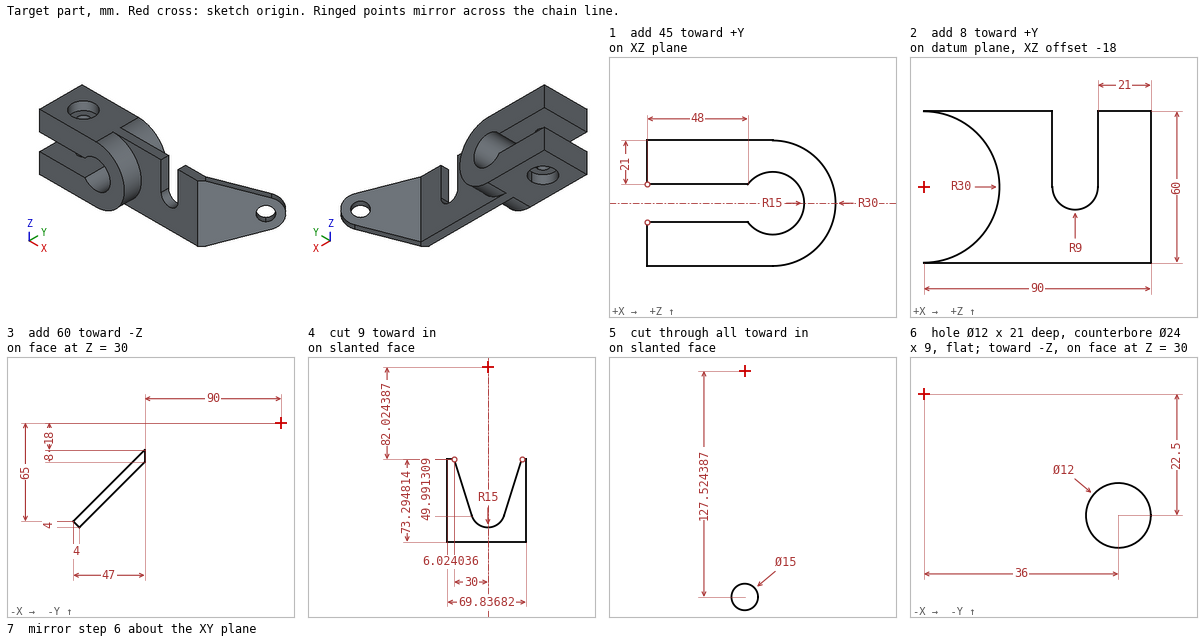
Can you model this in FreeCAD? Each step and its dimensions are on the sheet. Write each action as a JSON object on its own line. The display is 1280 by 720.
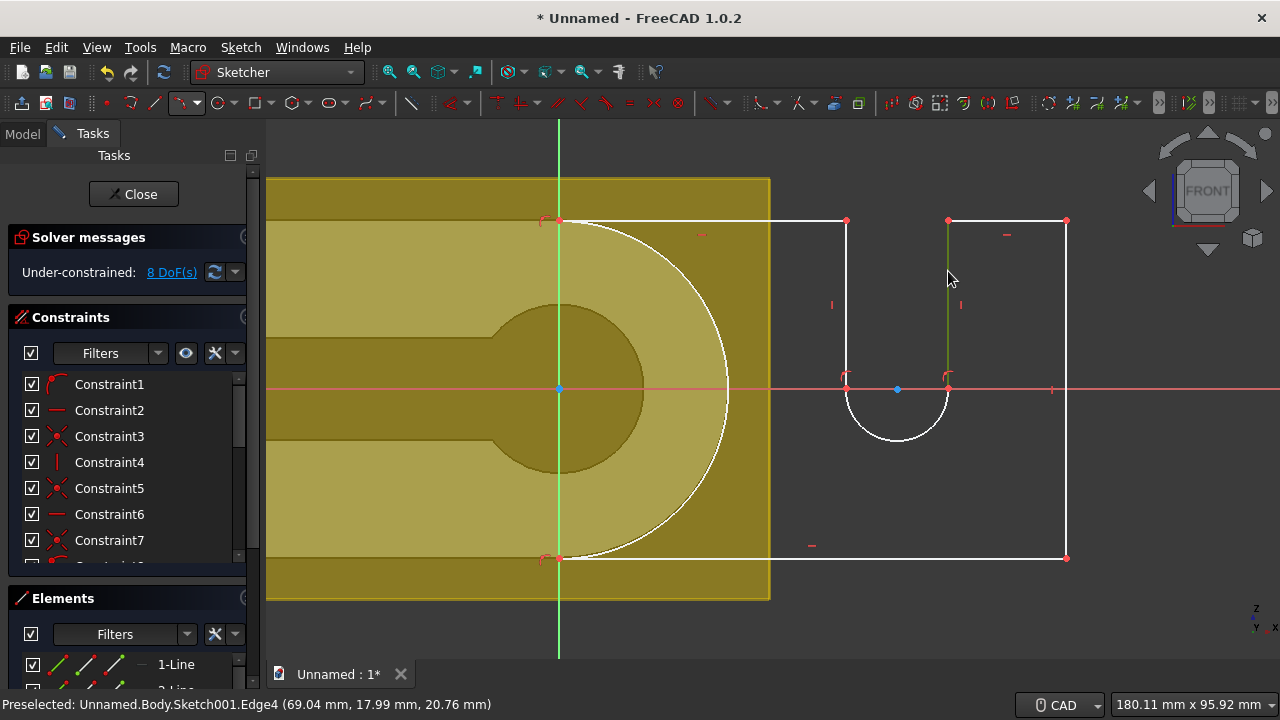
{"action": "left_click", "coordinate": [867, 431]}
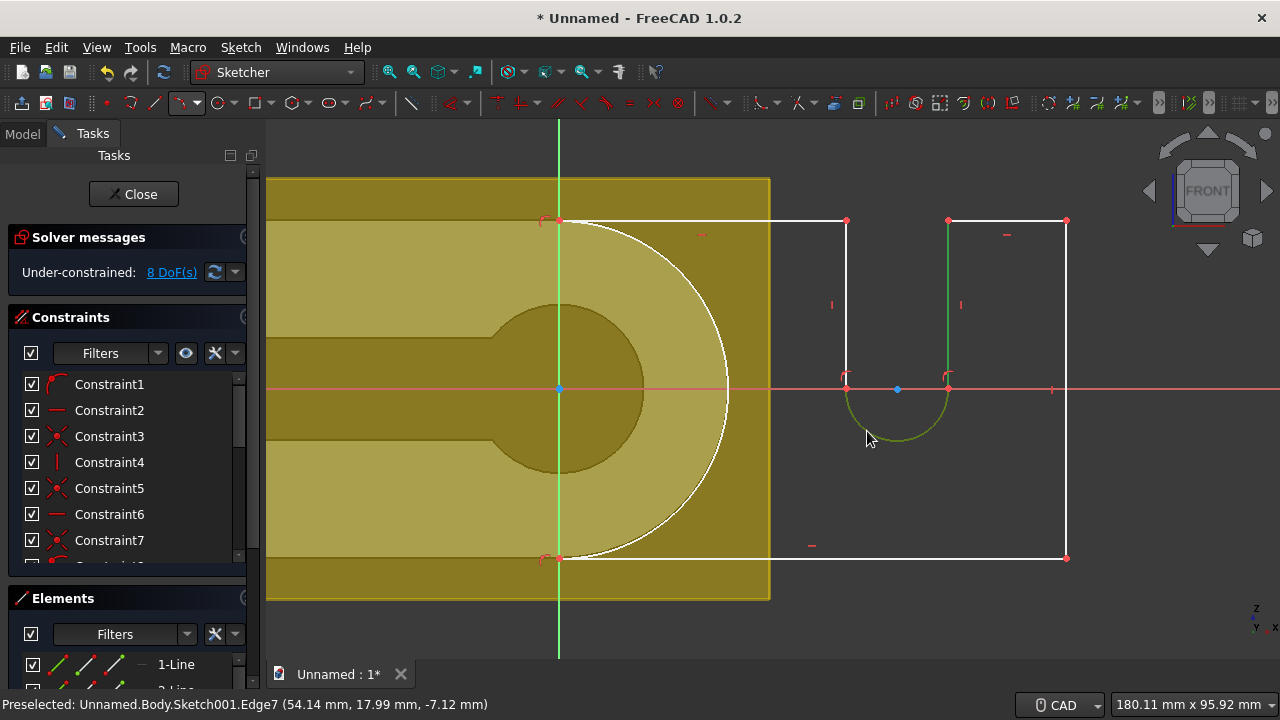
{"action": "left_click", "coordinate": [606, 104]}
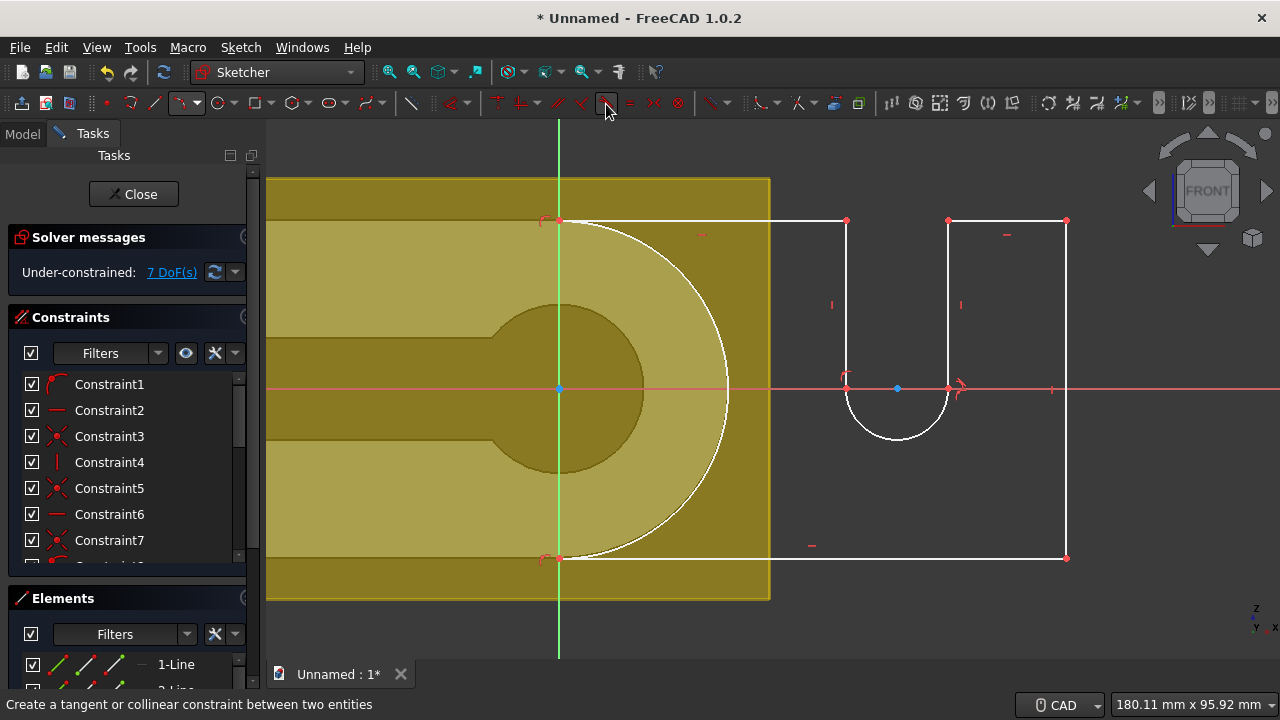
{"action": "left_click_drag", "start_coordinate": [549, 379], "coordinate": [569, 400]}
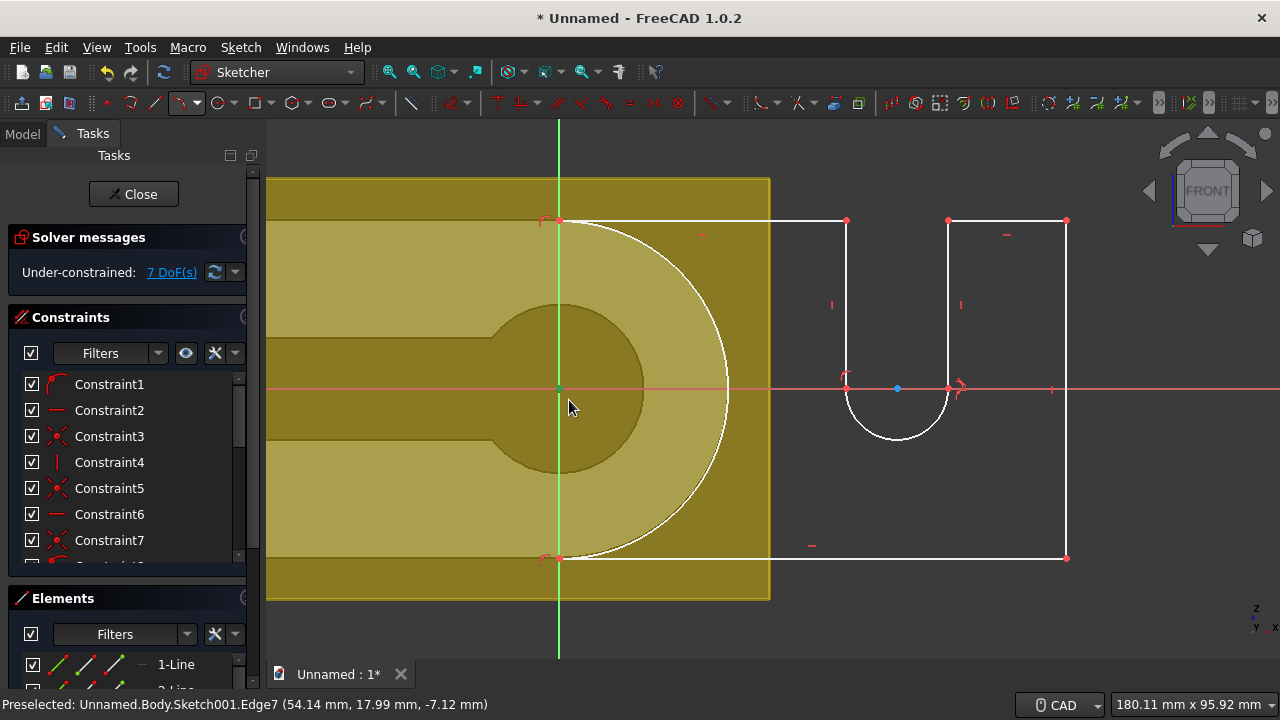
{"action": "left_click", "coordinate": [498, 104]}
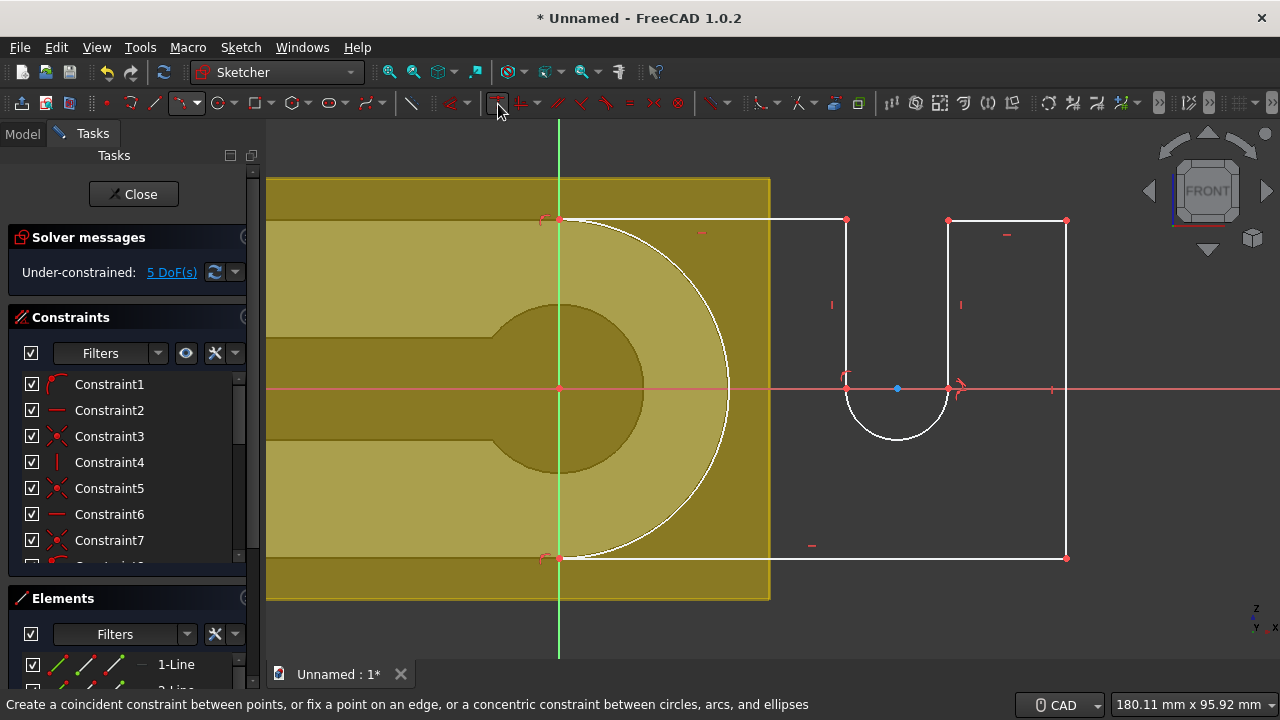
{"action": "left_click", "coordinate": [450, 104]}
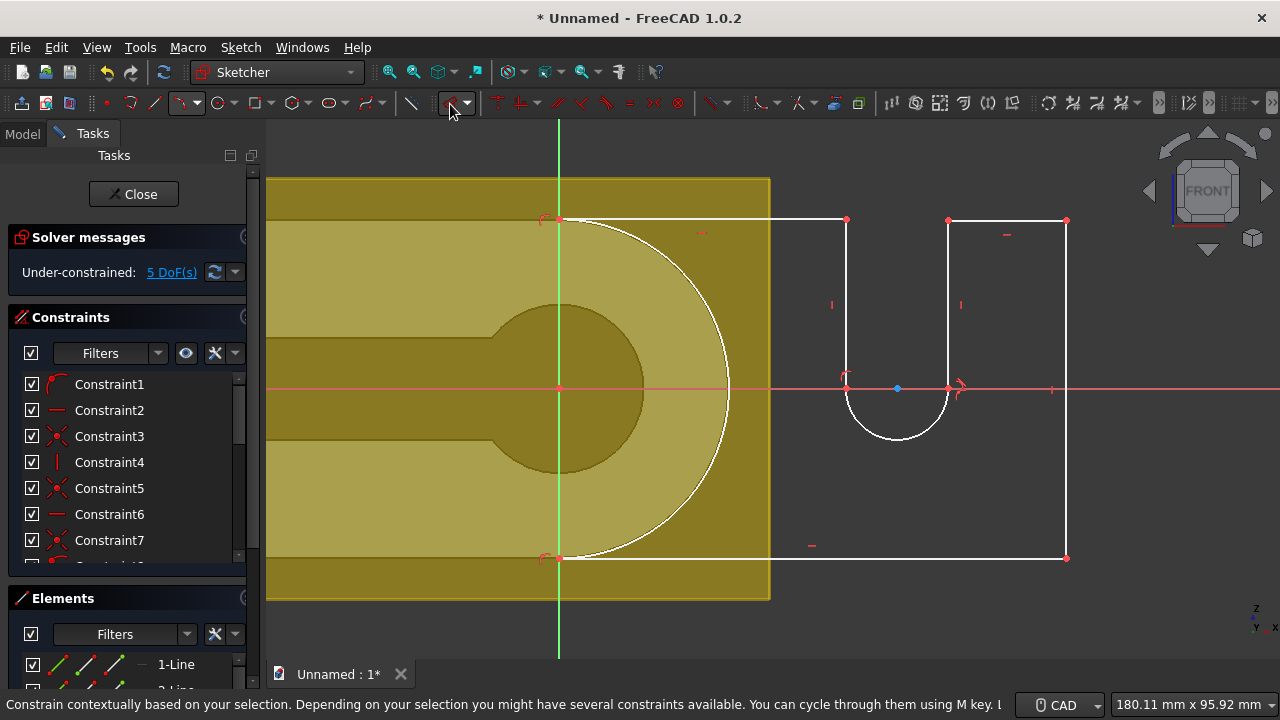
{"action": "left_click", "coordinate": [867, 430]}
{"action": "left_click", "coordinate": [848, 456]}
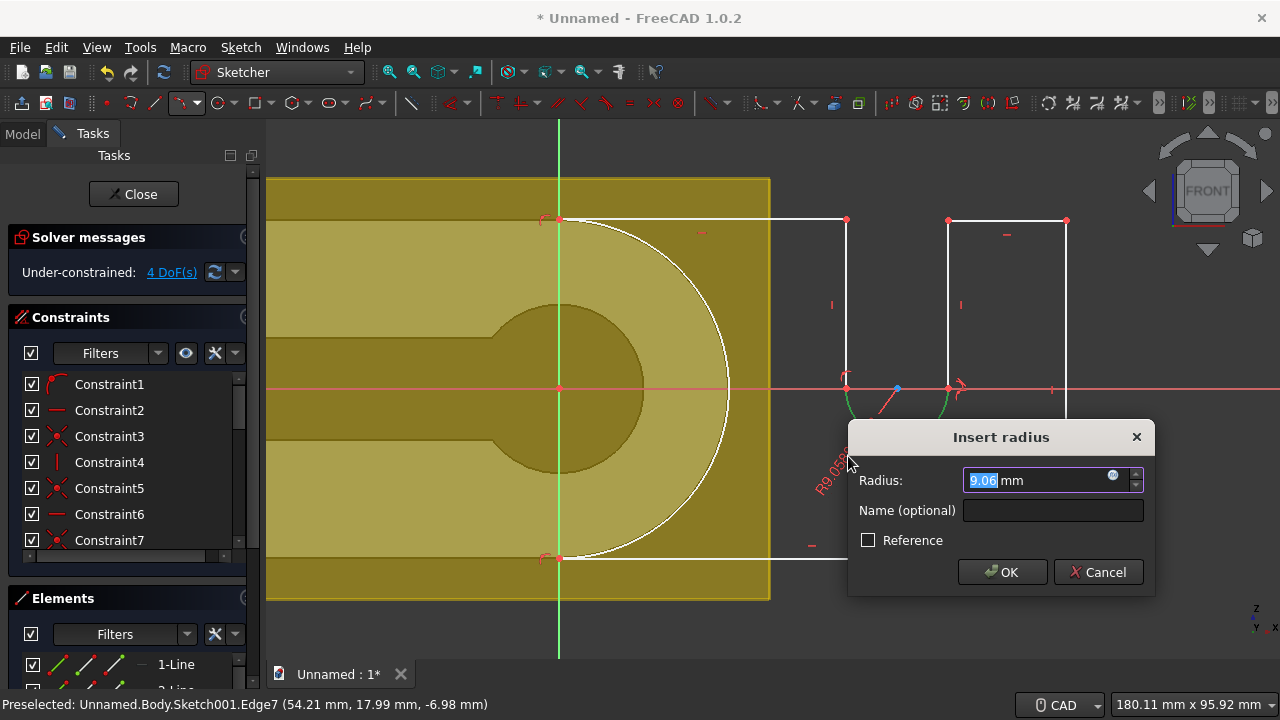
{"action": "type", "text": "9"}
{"action": "key", "text": "Return"}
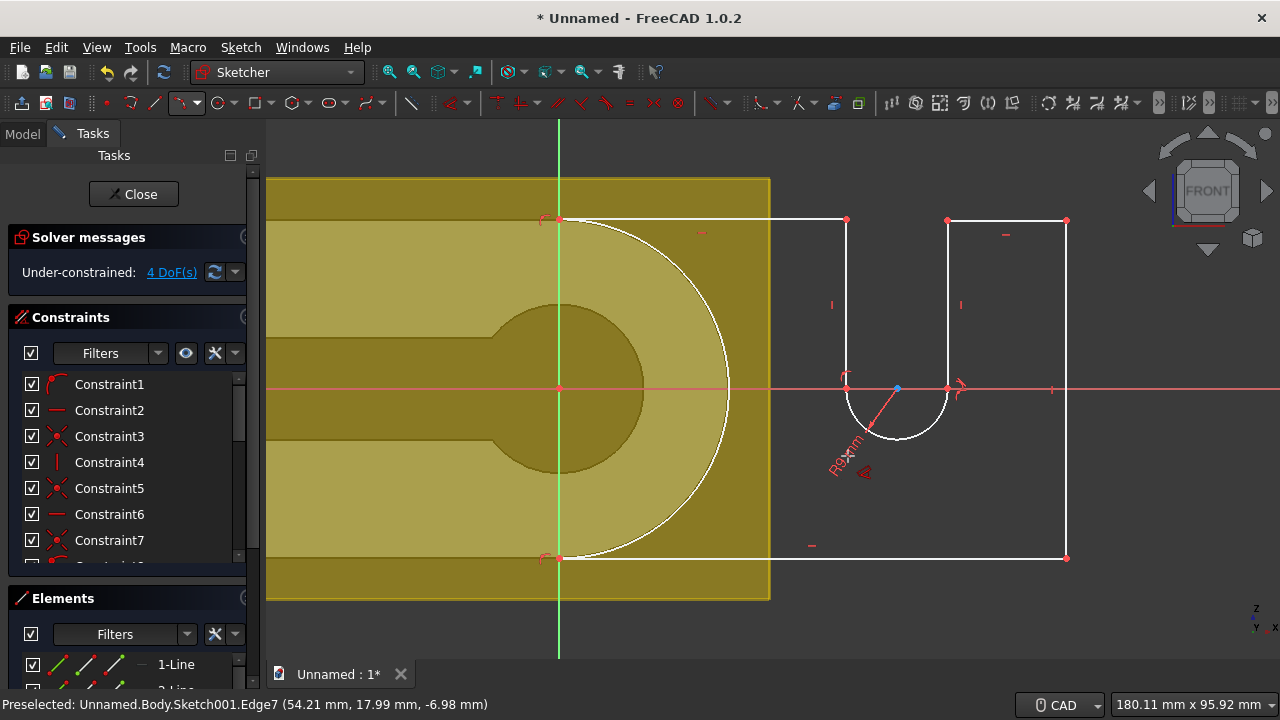
{"action": "left_click", "coordinate": [697, 489]}
{"action": "left_click", "coordinate": [723, 508]}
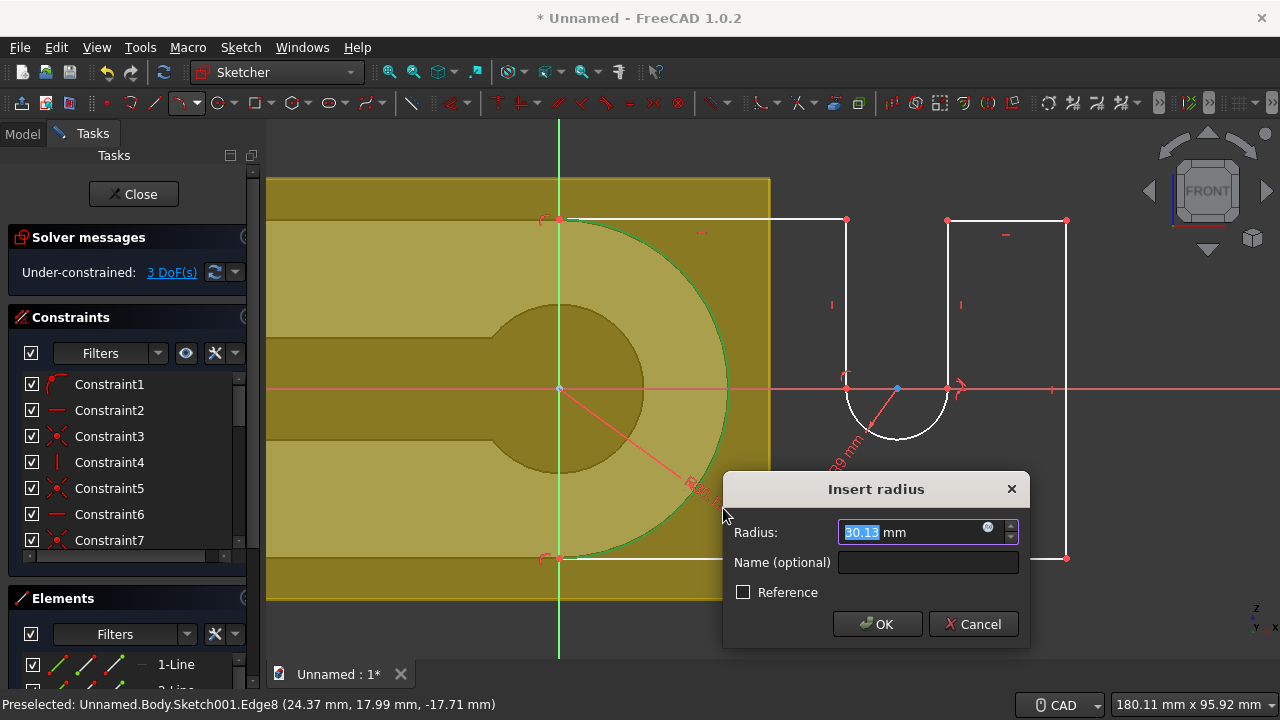
{"action": "type", "text": "30"}
{"action": "key", "text": "Return"}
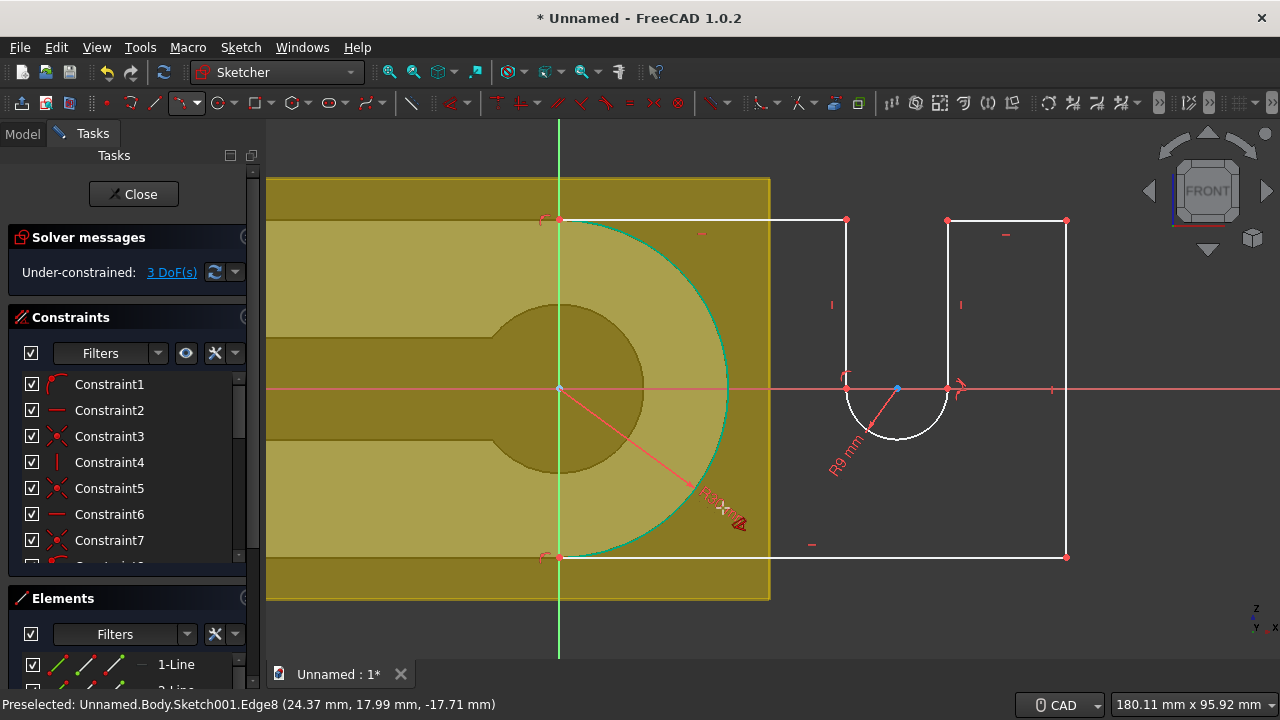
{"action": "left_click", "coordinate": [711, 558]}
{"action": "left_click", "coordinate": [813, 592]}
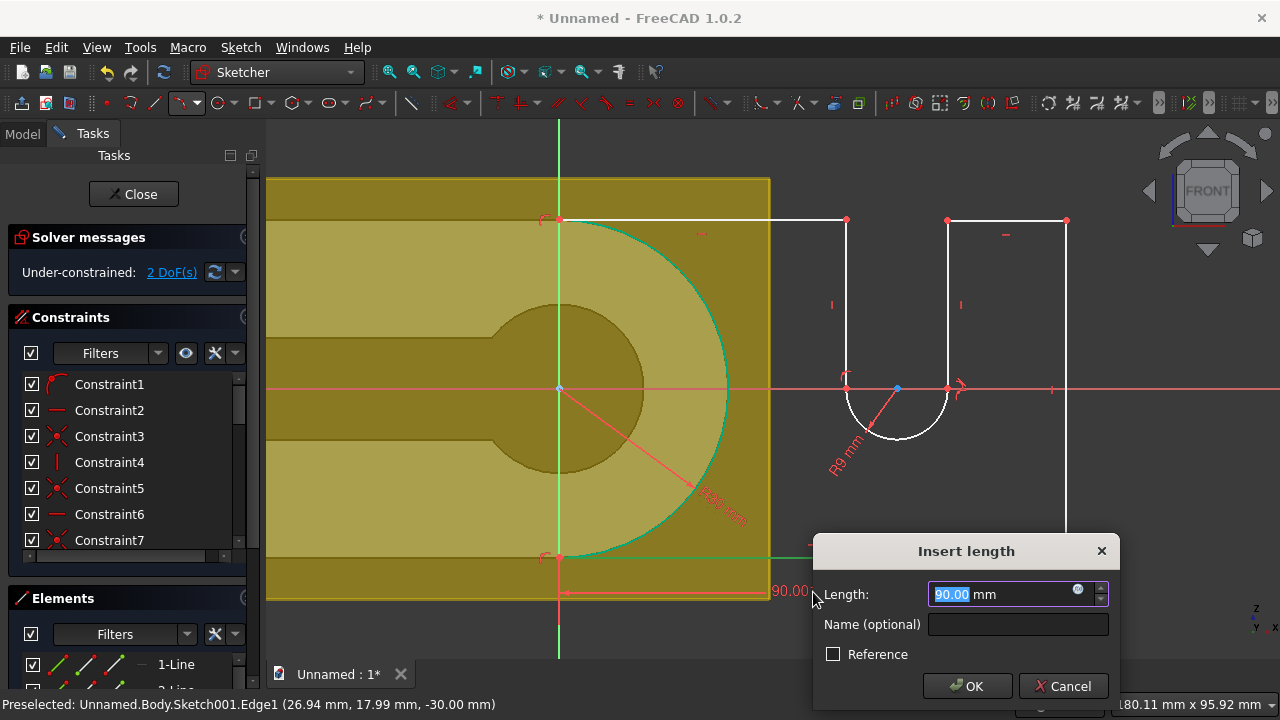
{"action": "type", "text": "90"}
{"action": "key", "text": "Return"}